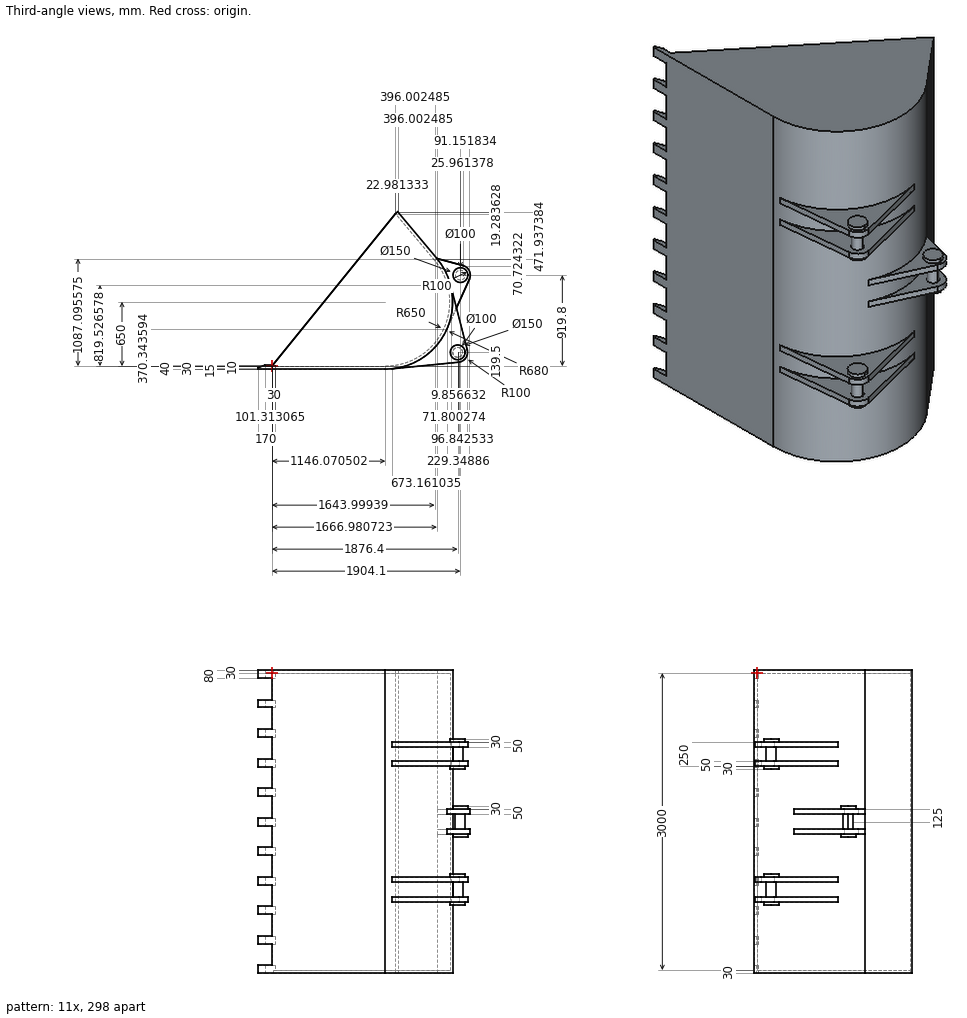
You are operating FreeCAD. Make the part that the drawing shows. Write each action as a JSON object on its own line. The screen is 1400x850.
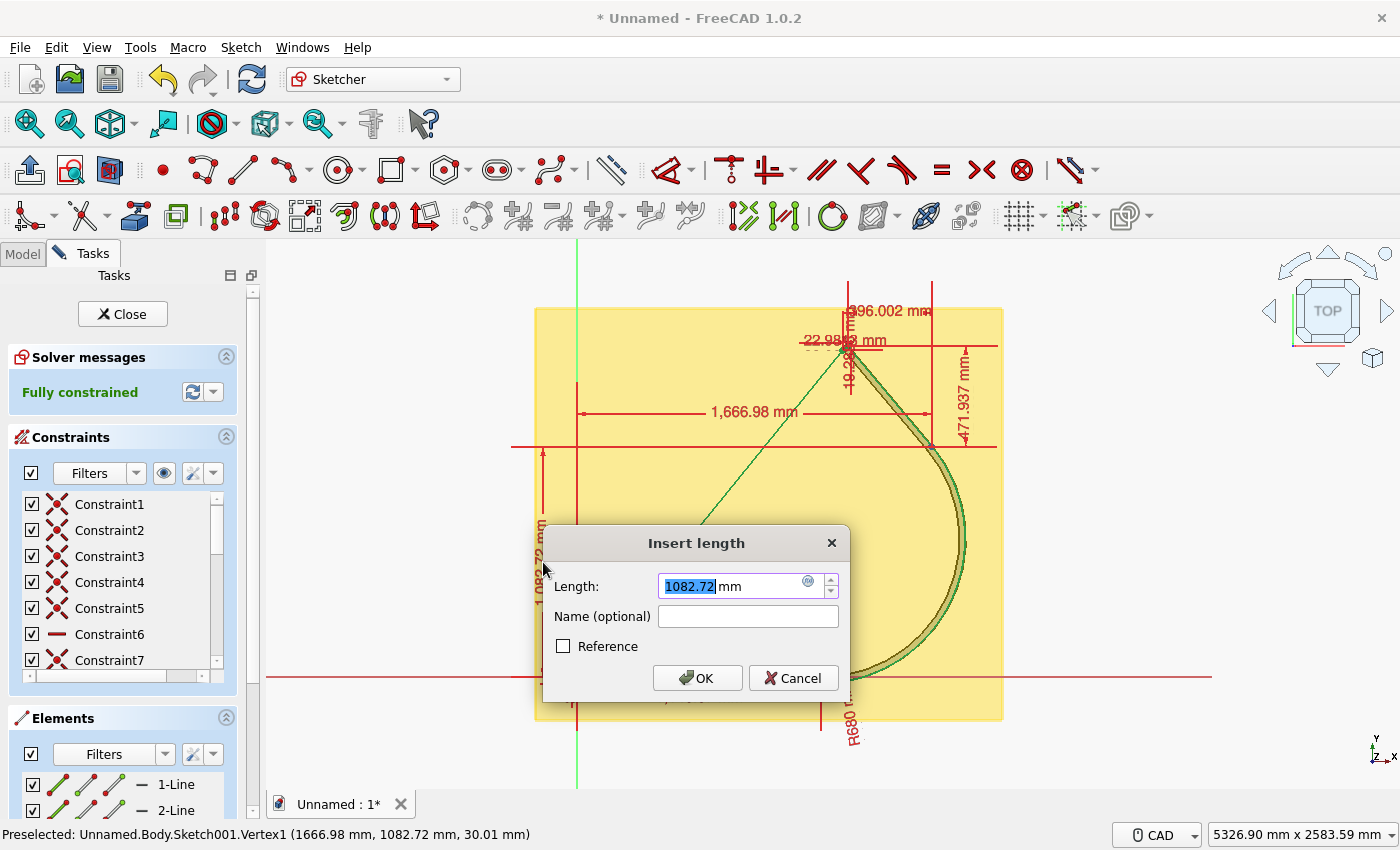
{"action": "type", "text": "1087.095575"}
{"action": "key", "text": "Return"}
{"action": "key", "text": "Escape"}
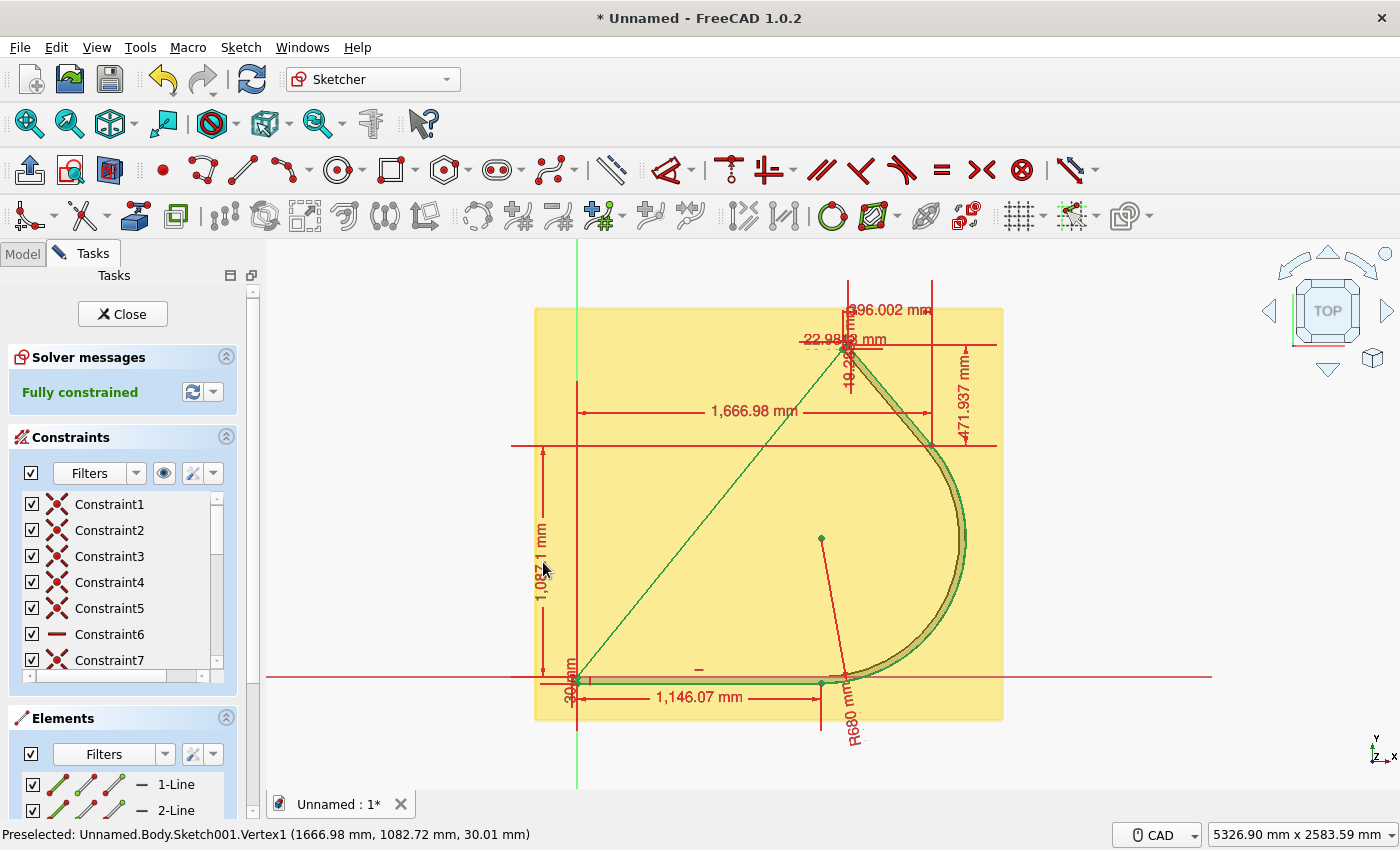
{"action": "left_click", "coordinate": [123, 314]}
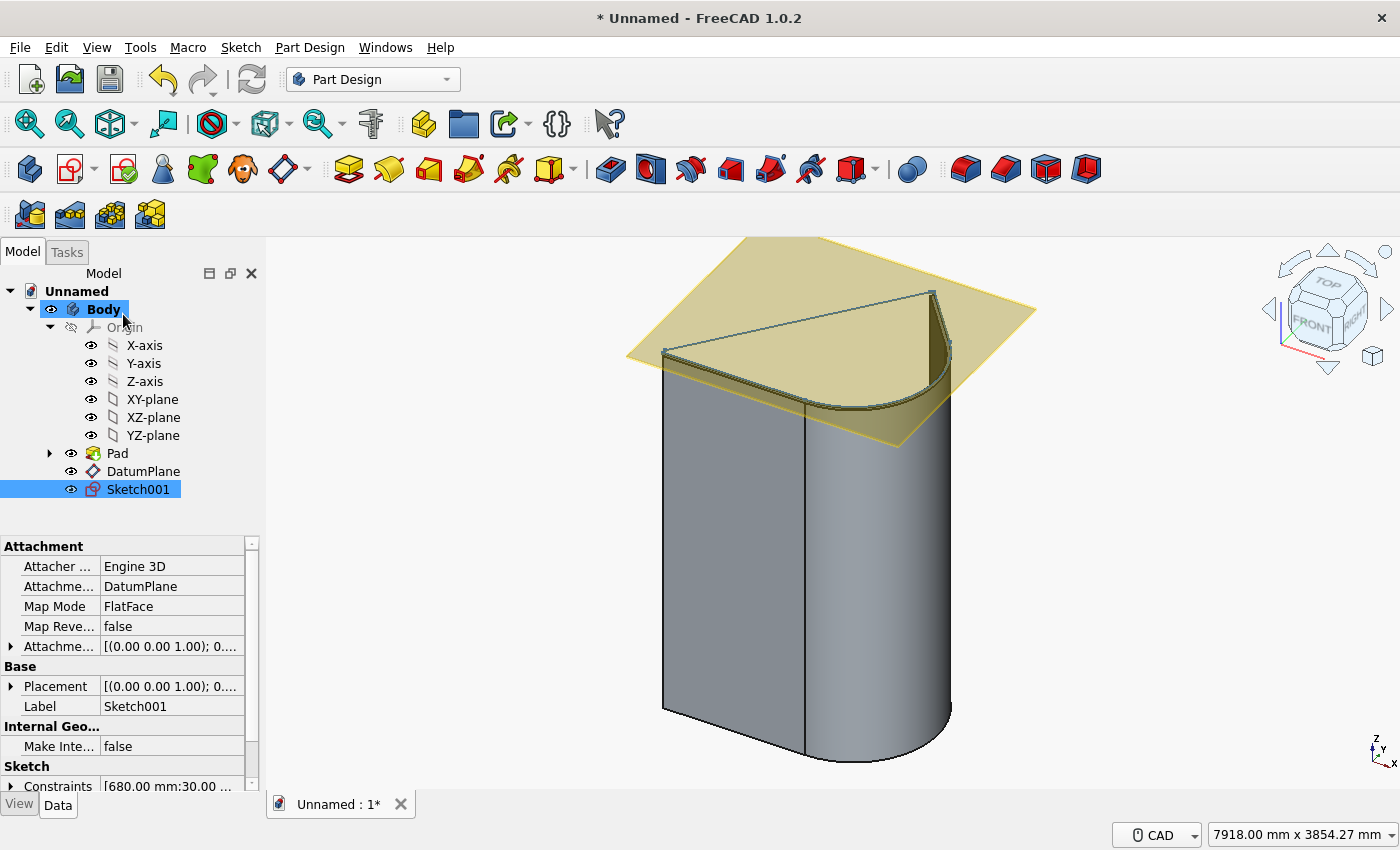
{"action": "left_click", "coordinate": [350, 170]}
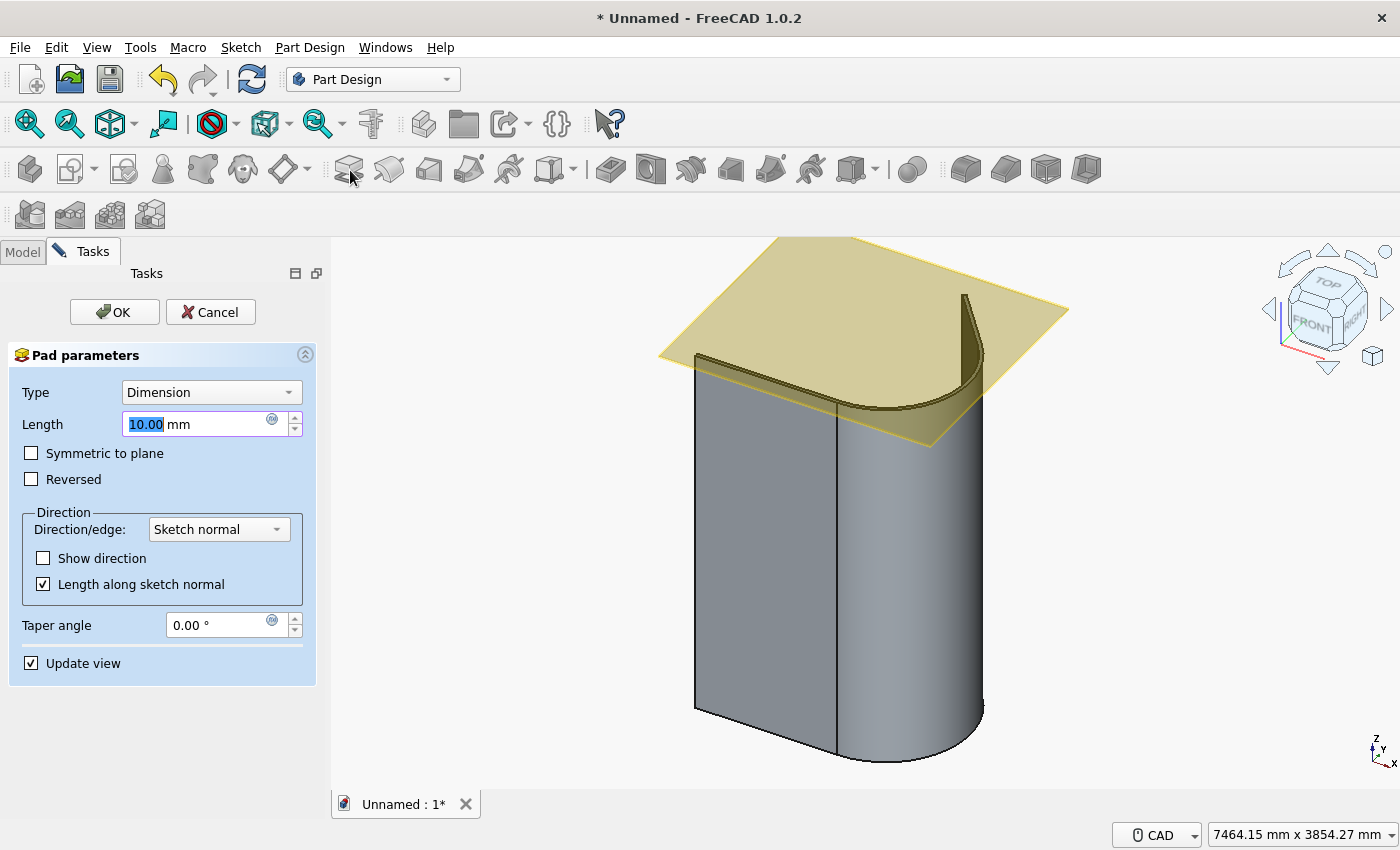
{"action": "type", "text": "30"}
{"action": "key", "text": "Tab"}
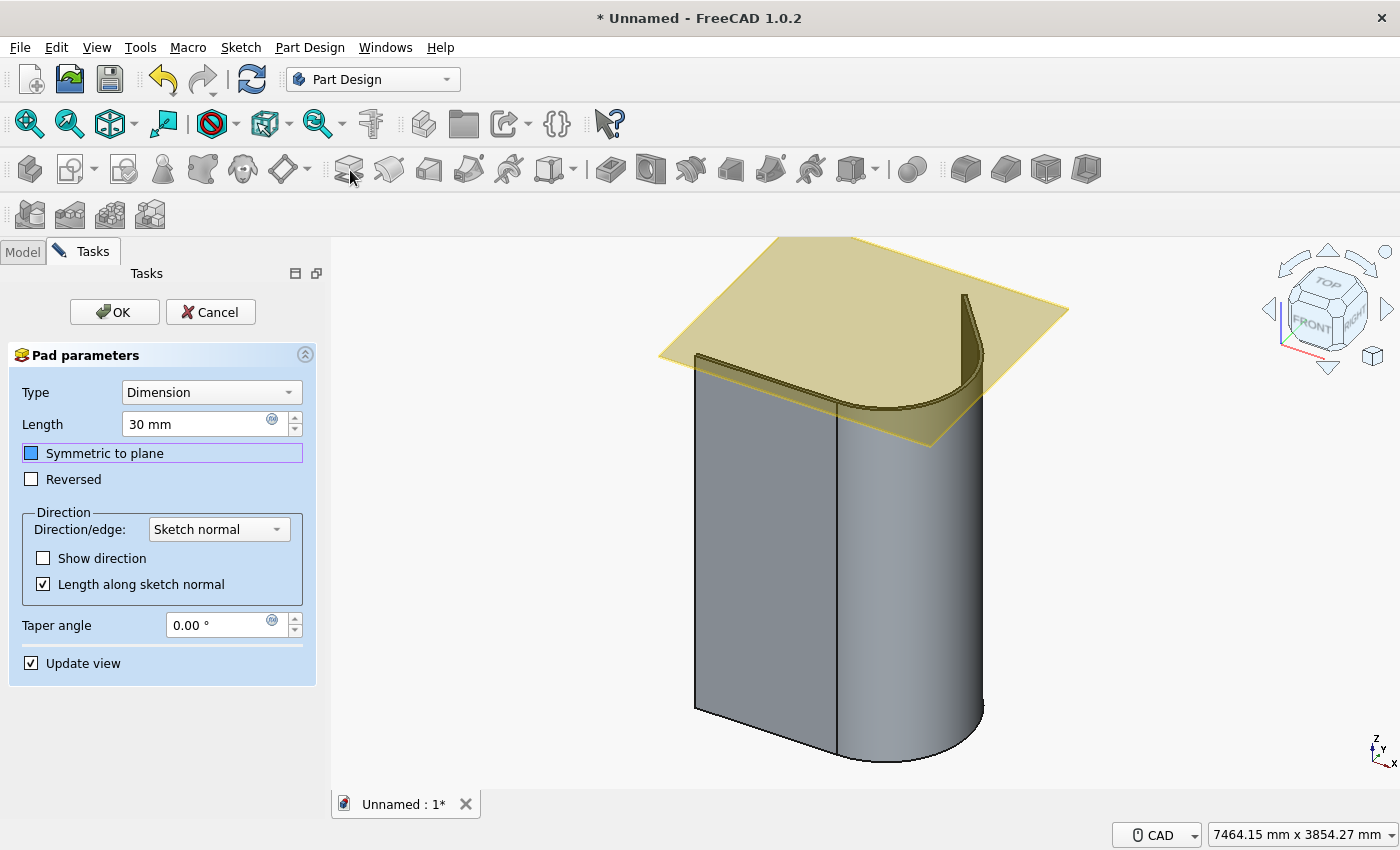
{"action": "left_click", "coordinate": [30, 479]}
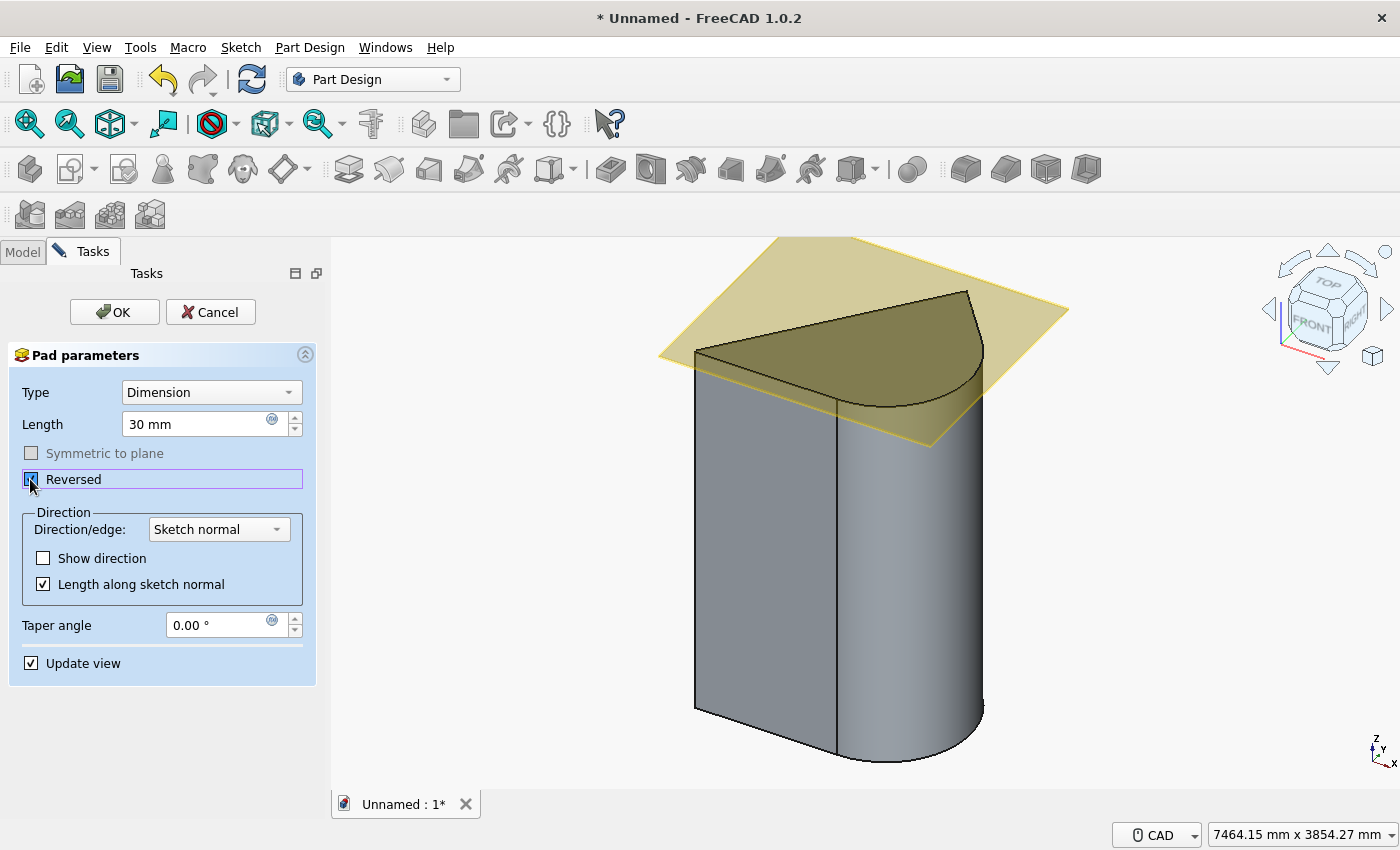
{"action": "left_click", "coordinate": [115, 312]}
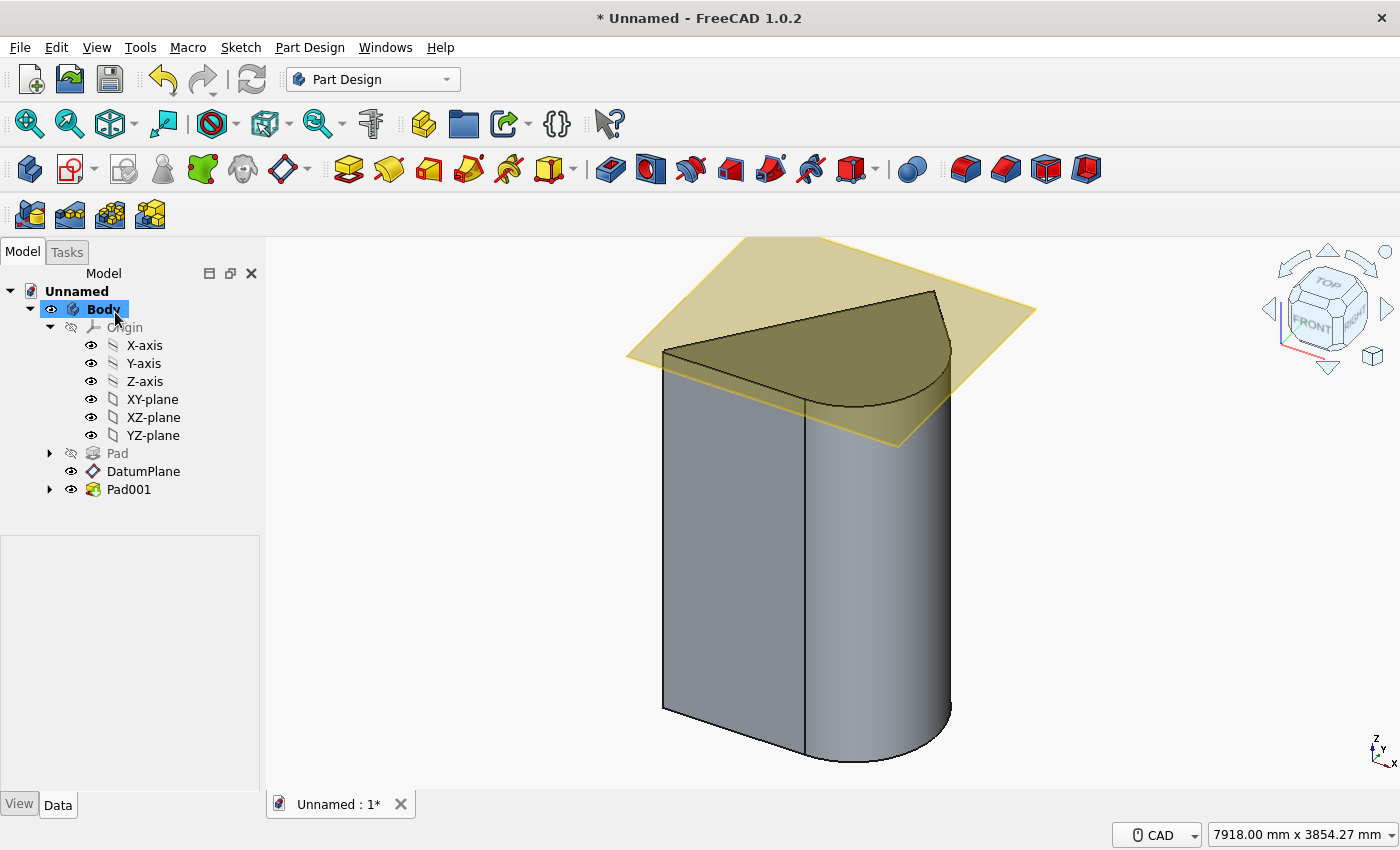
{"action": "left_click", "coordinate": [116, 471]}
{"action": "key", "text": "space"}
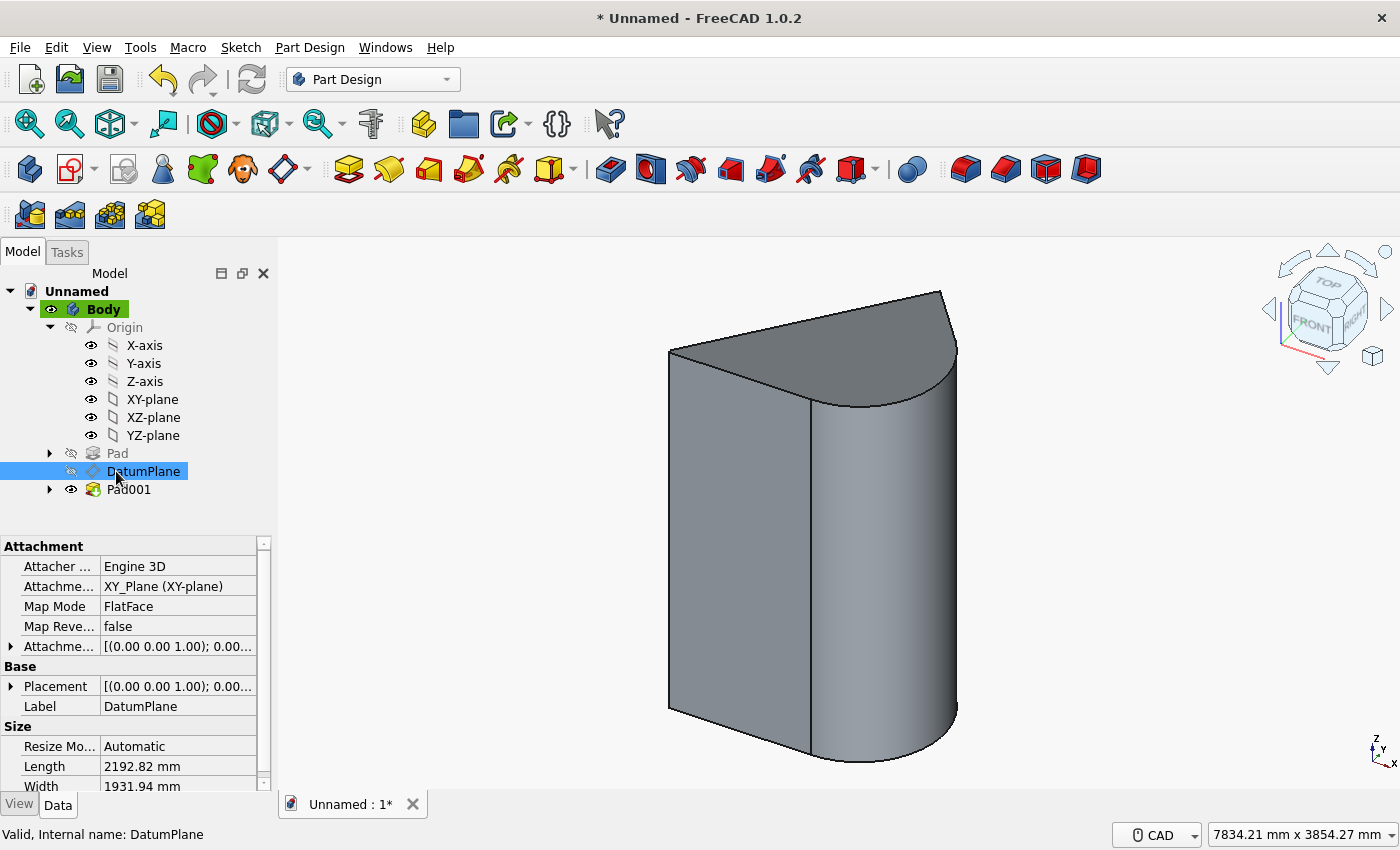
{"action": "key", "text": "5"}